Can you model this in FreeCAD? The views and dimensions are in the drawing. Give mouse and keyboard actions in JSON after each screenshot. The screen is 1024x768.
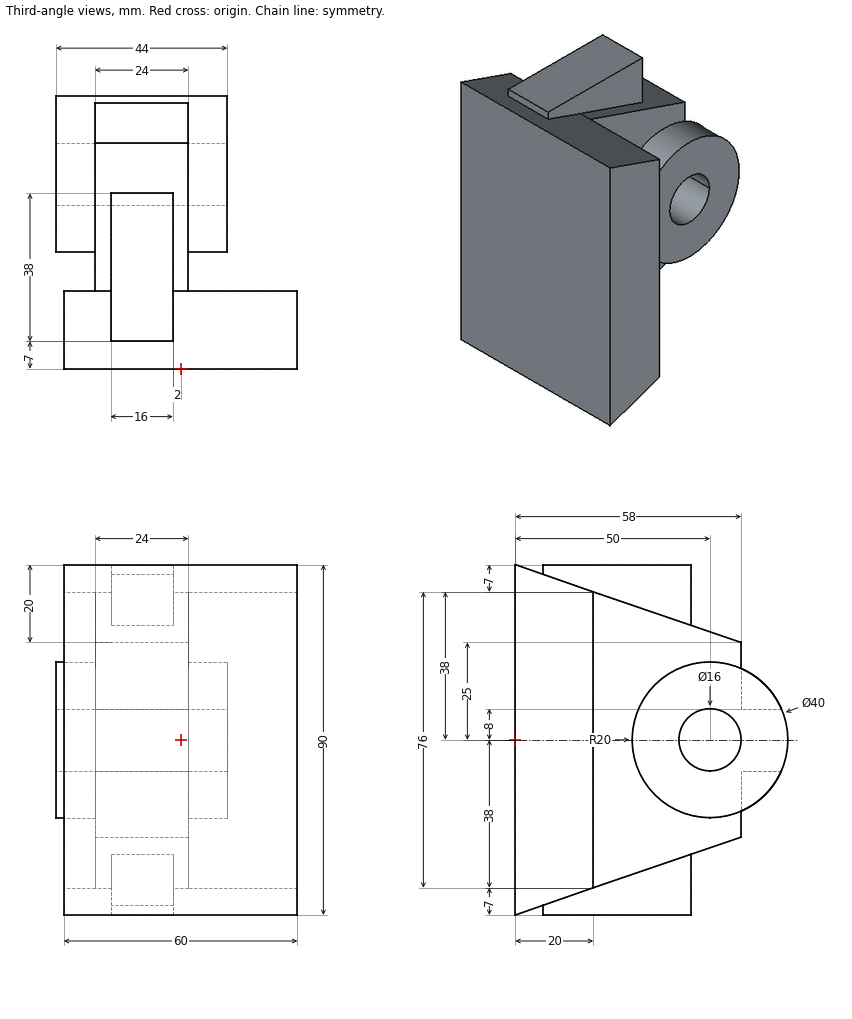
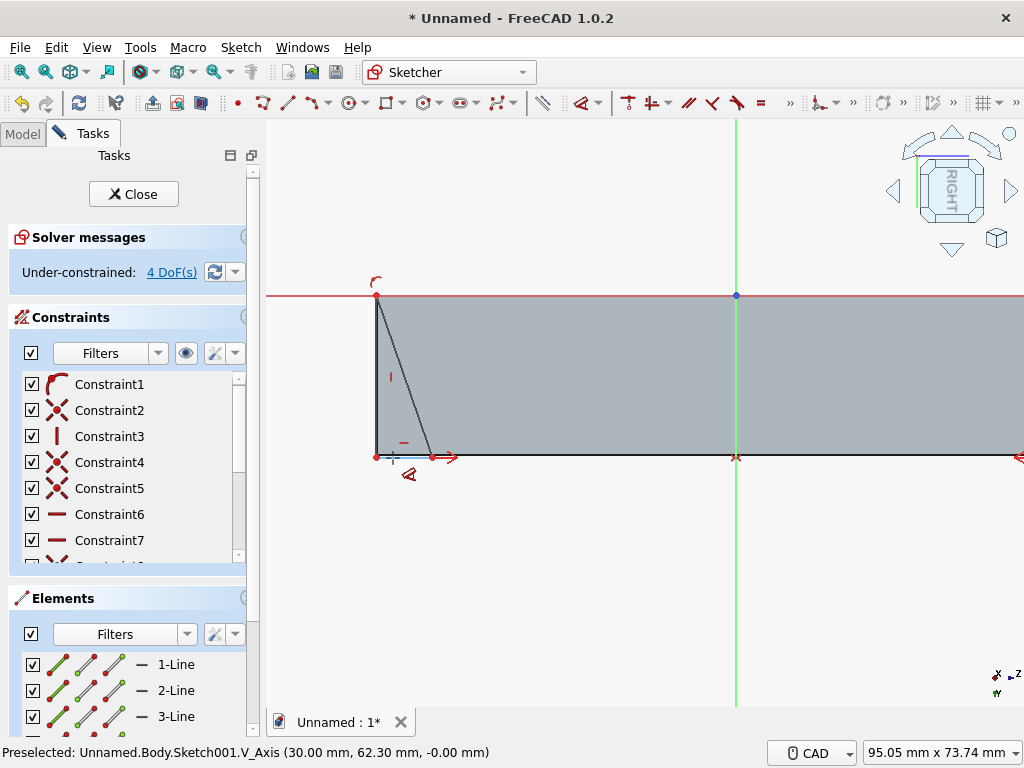
{"action": "left_click", "coordinate": [393, 458]}
{"action": "left_click", "coordinate": [404, 492]}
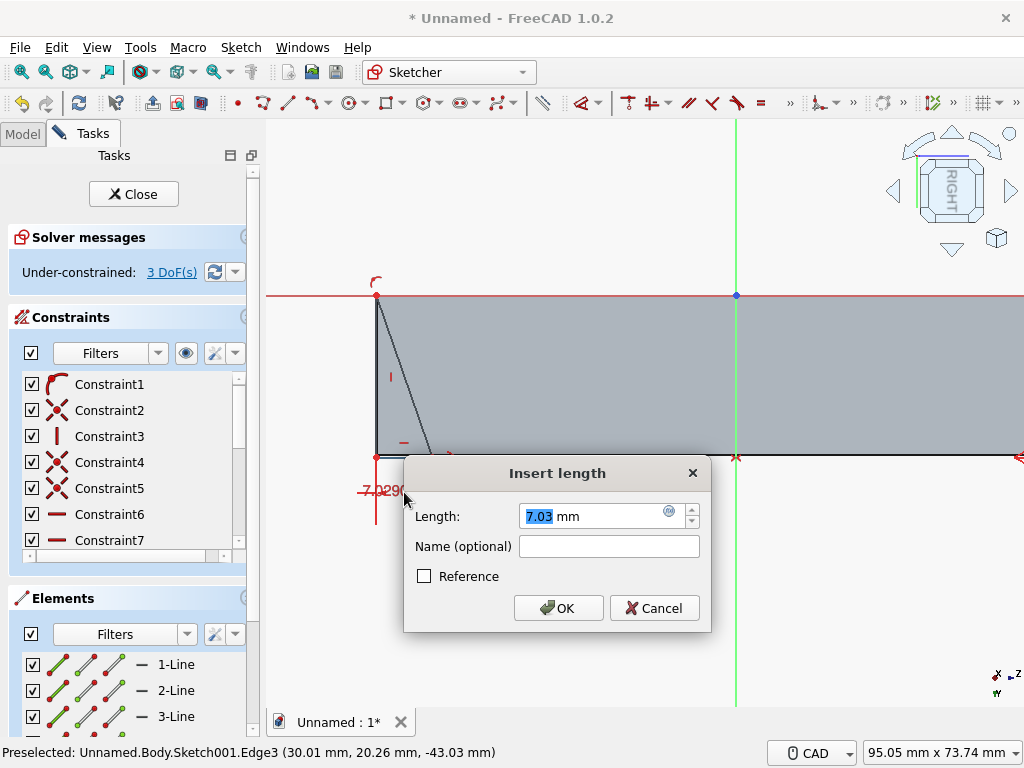
{"action": "type", "text": "7"}
{"action": "key", "text": "Return"}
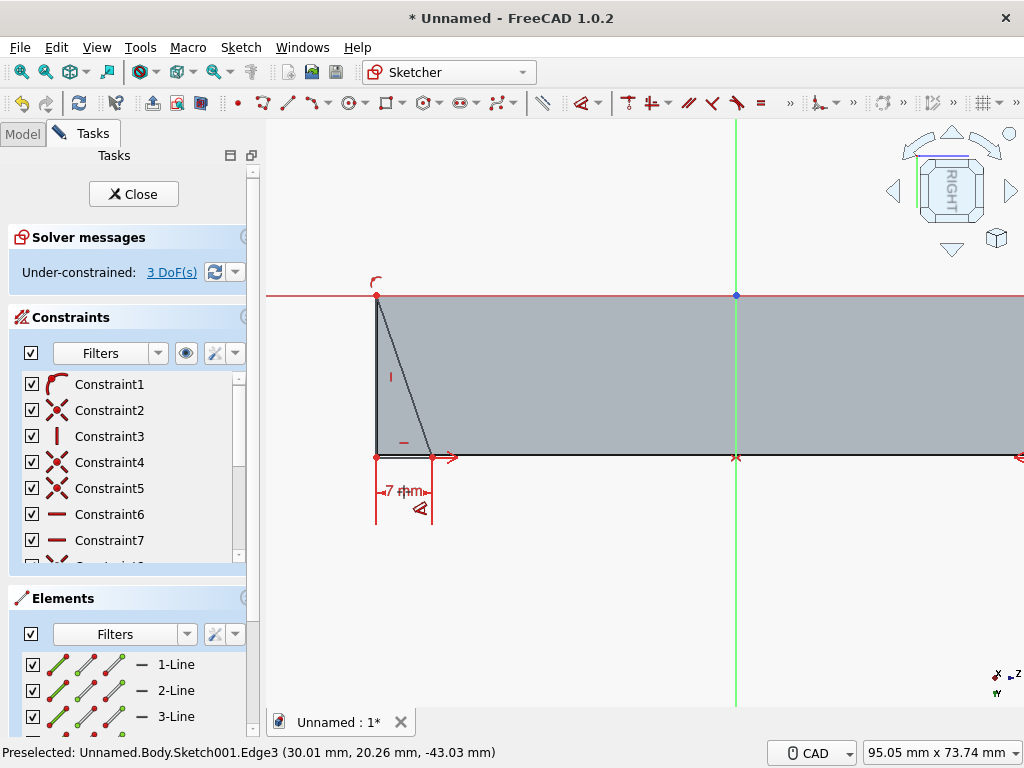
{"action": "scroll", "coordinate": [382, 458], "scroll_direction": "down", "scroll_amount": 3}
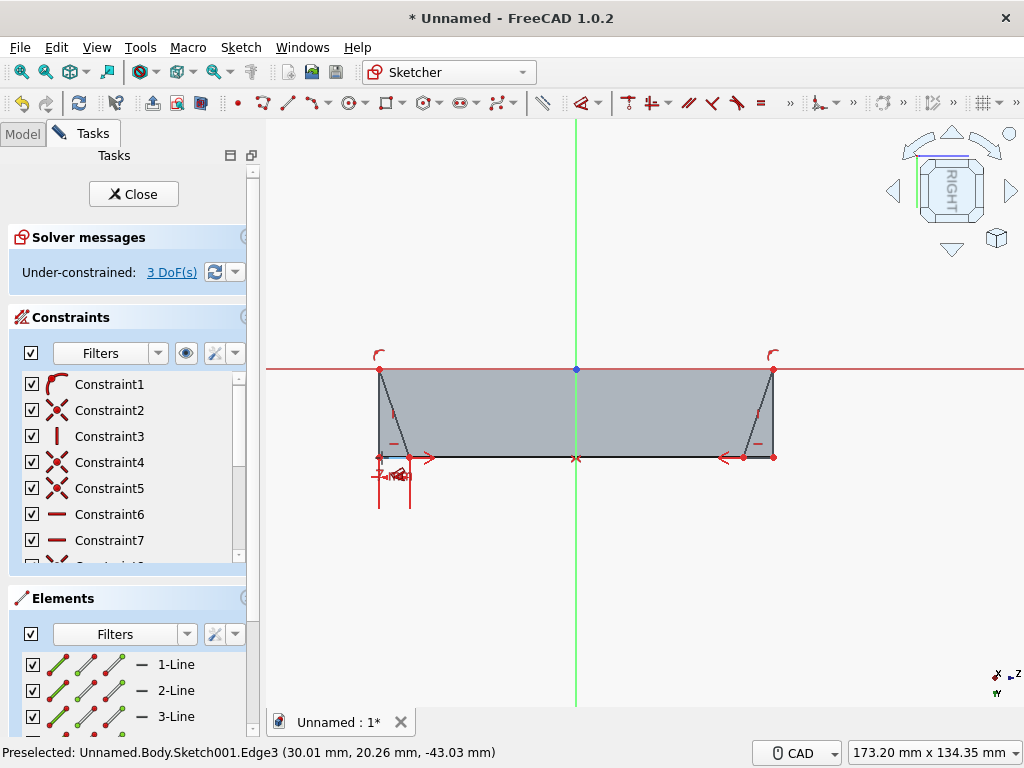
{"action": "scroll", "coordinate": [752, 458], "scroll_direction": "up", "scroll_amount": 3}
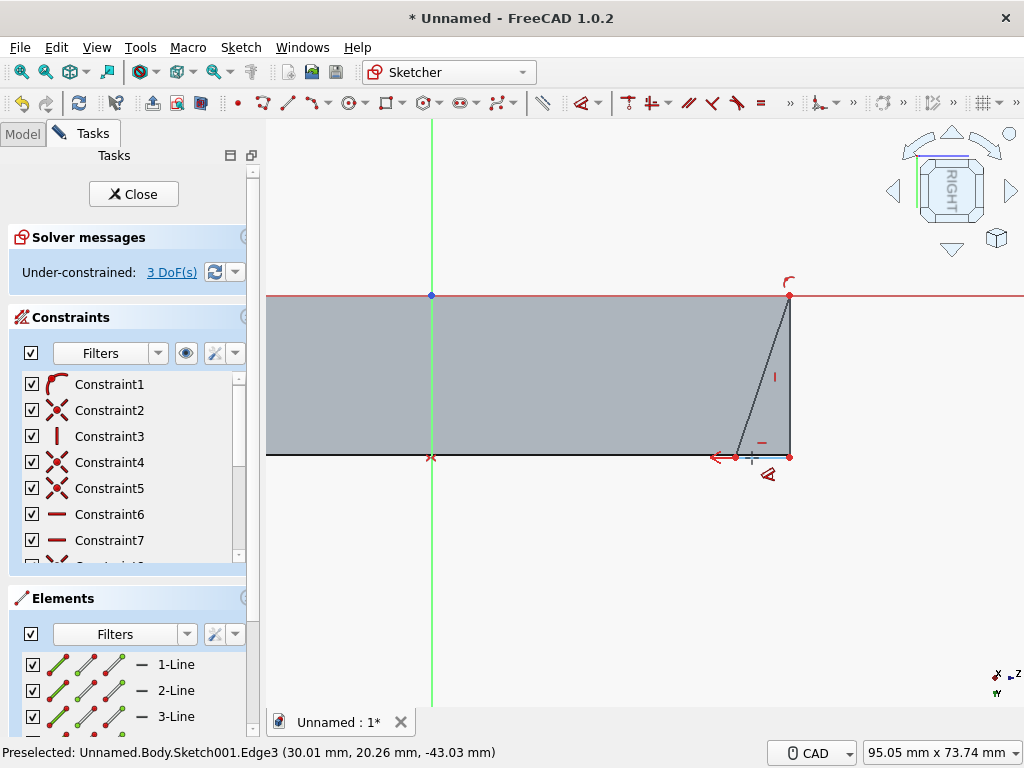
{"action": "left_click", "coordinate": [752, 458]}
{"action": "left_click", "coordinate": [763, 492]}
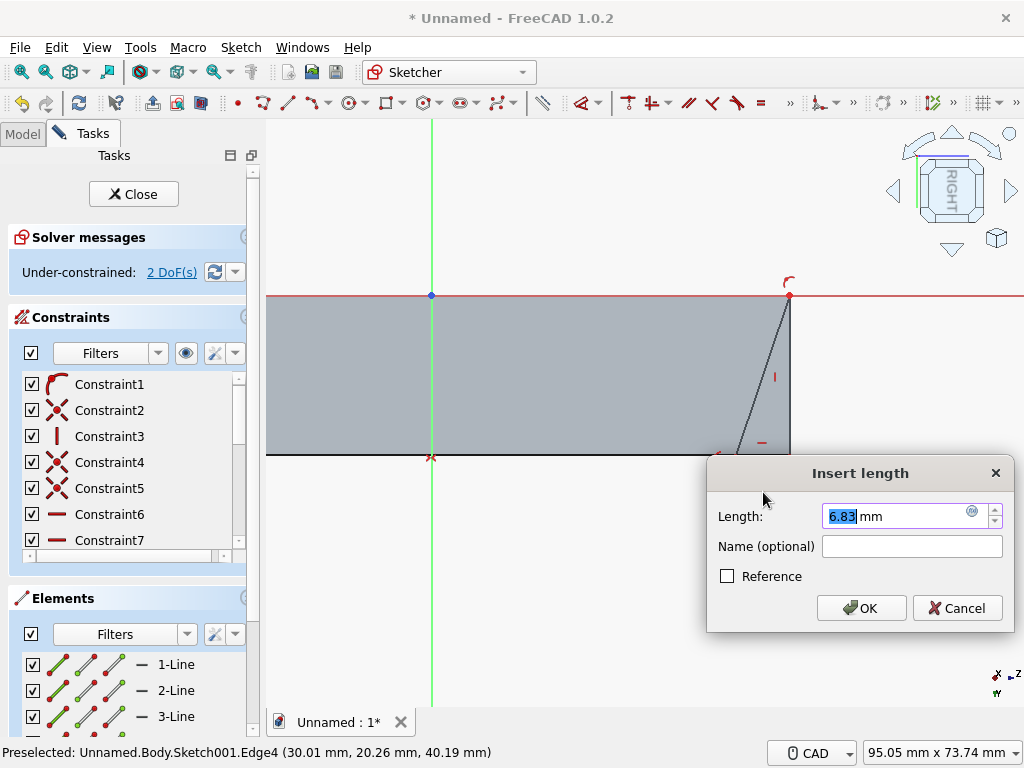
{"action": "type", "text": "7"}
{"action": "key", "text": "Return"}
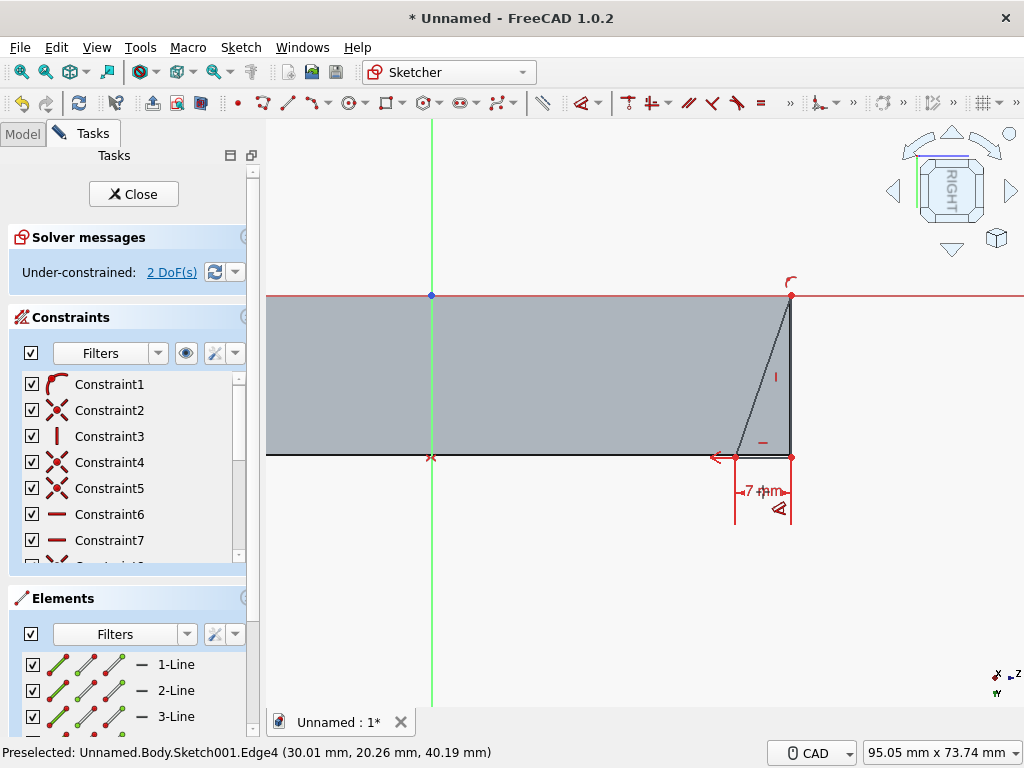
{"action": "scroll", "coordinate": [753, 458], "scroll_direction": "down", "scroll_amount": 3}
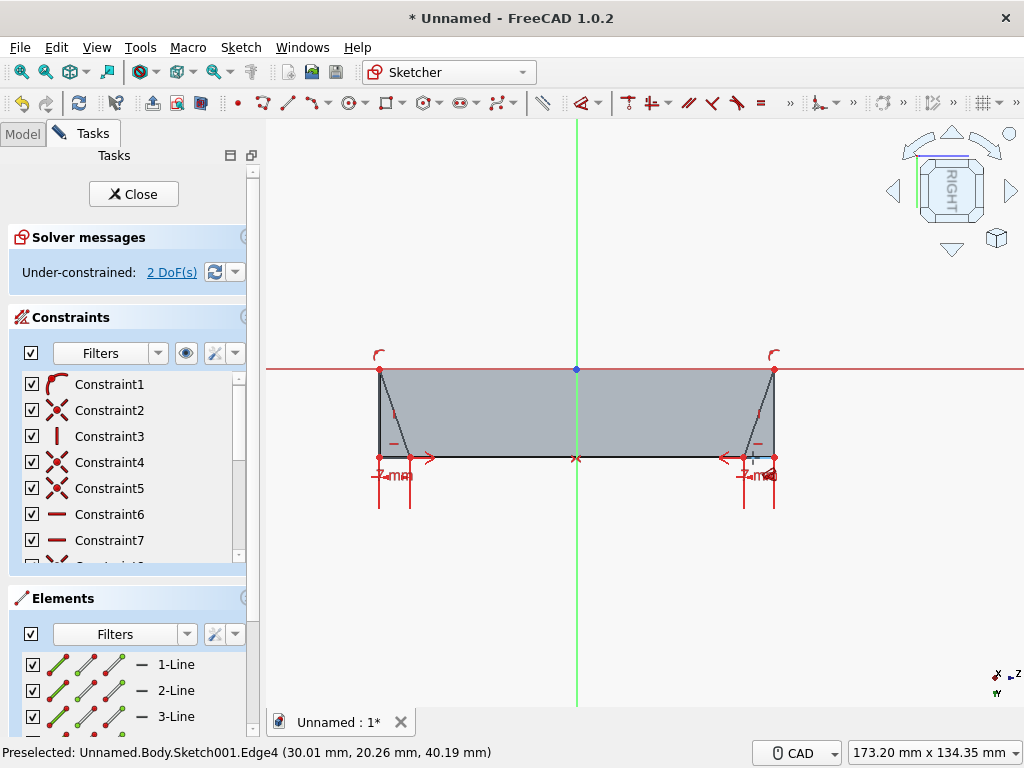
{"action": "scroll", "coordinate": [379, 396], "scroll_direction": "up", "scroll_amount": 3}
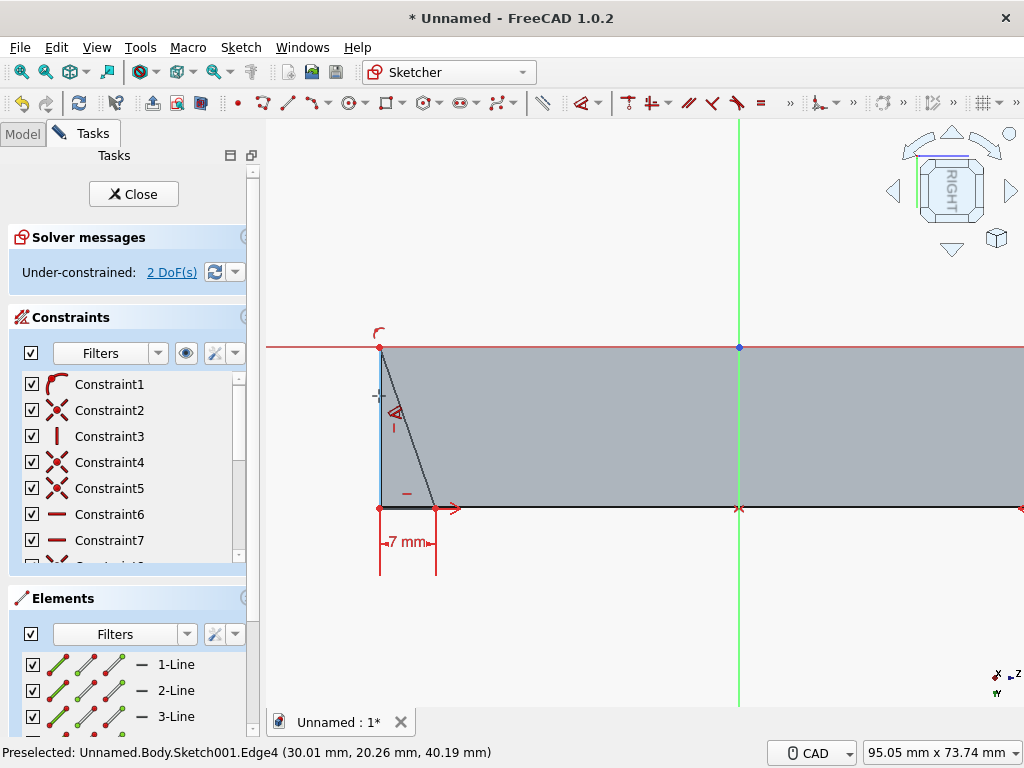
{"action": "left_click", "coordinate": [380, 395]}
{"action": "left_click", "coordinate": [346, 428]}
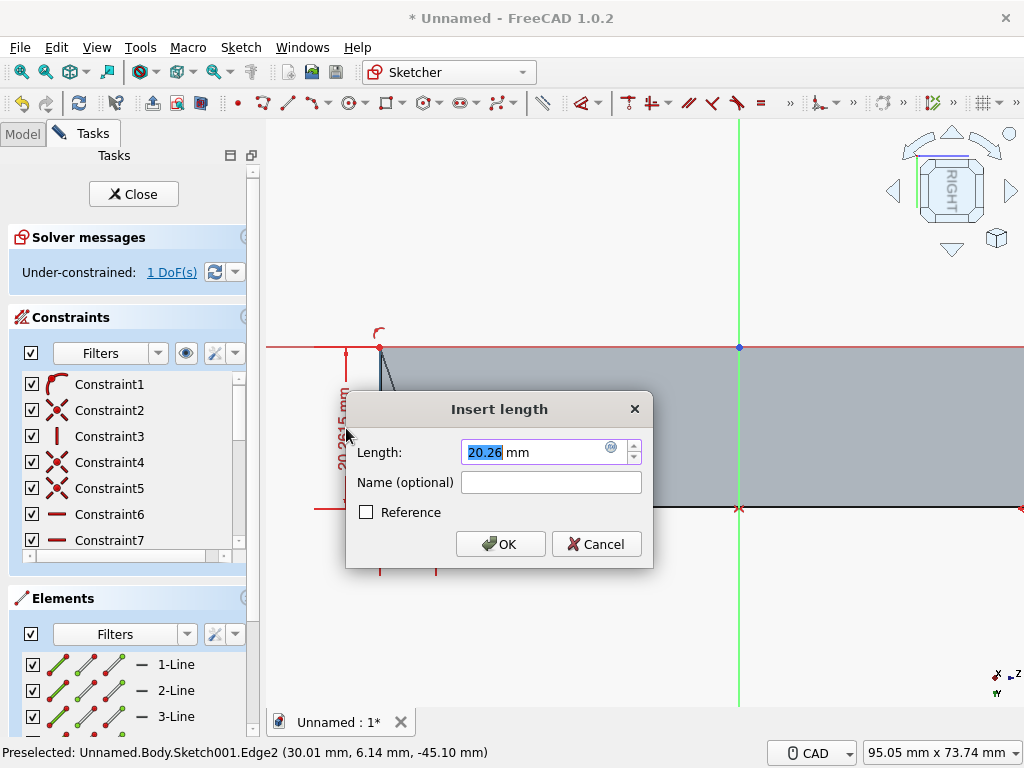
{"action": "type", "text": "20"}
{"action": "key", "text": "Return"}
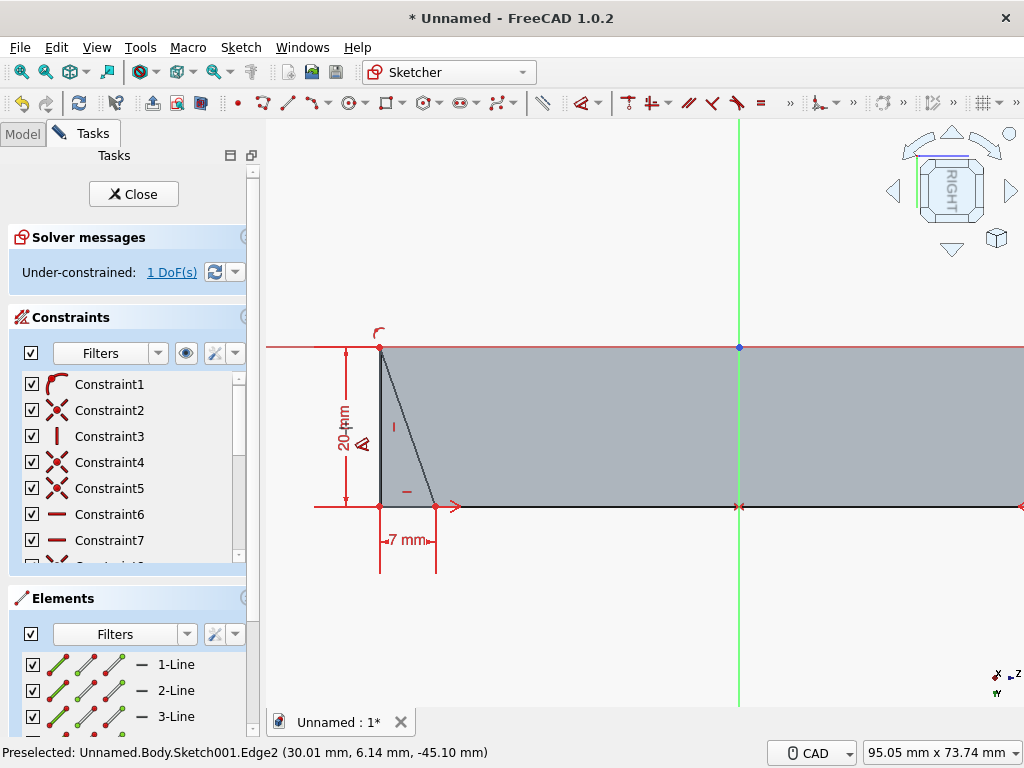
{"action": "left_click", "coordinate": [436, 506]}
{"action": "left_click", "coordinate": [587, 540]}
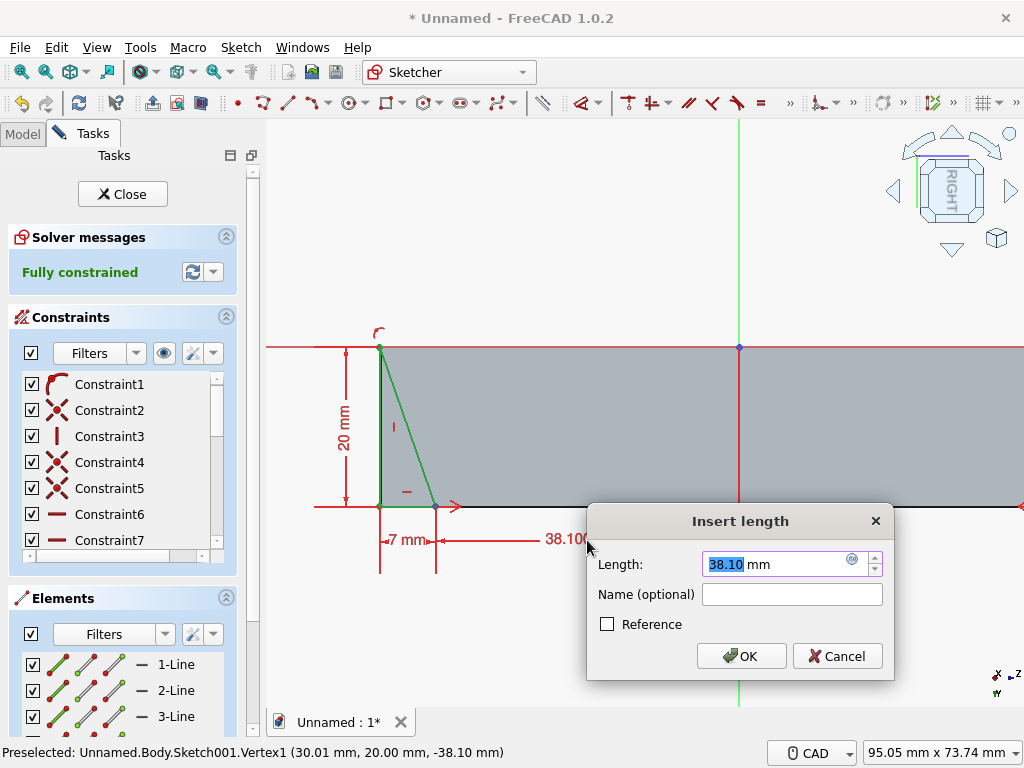
{"action": "type", "text": "38"}
{"action": "key", "text": "Return"}
{"action": "key", "text": "Escape"}